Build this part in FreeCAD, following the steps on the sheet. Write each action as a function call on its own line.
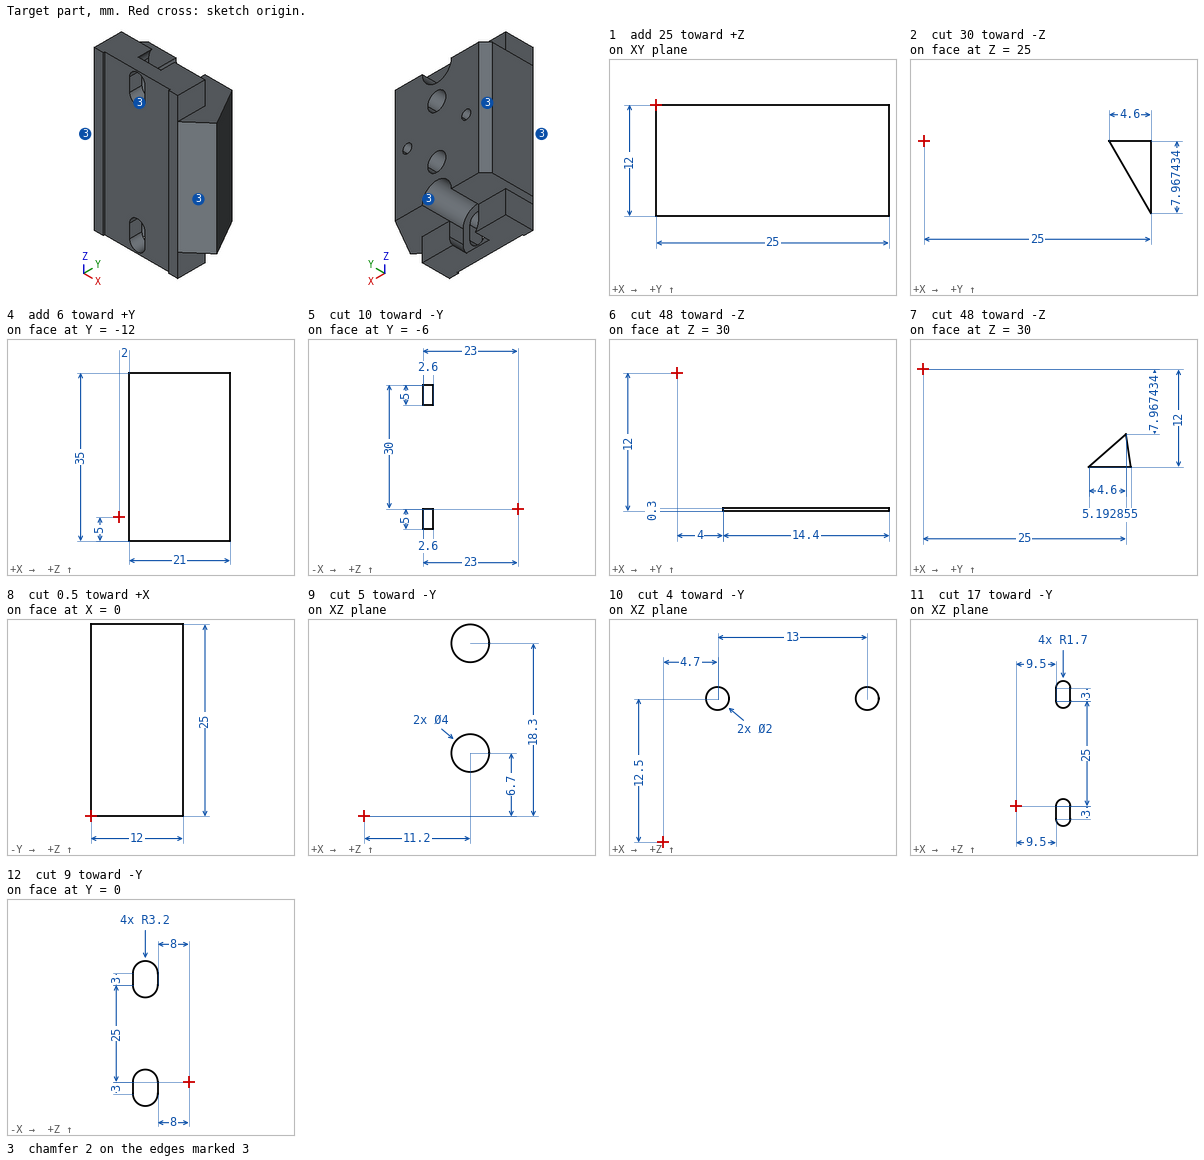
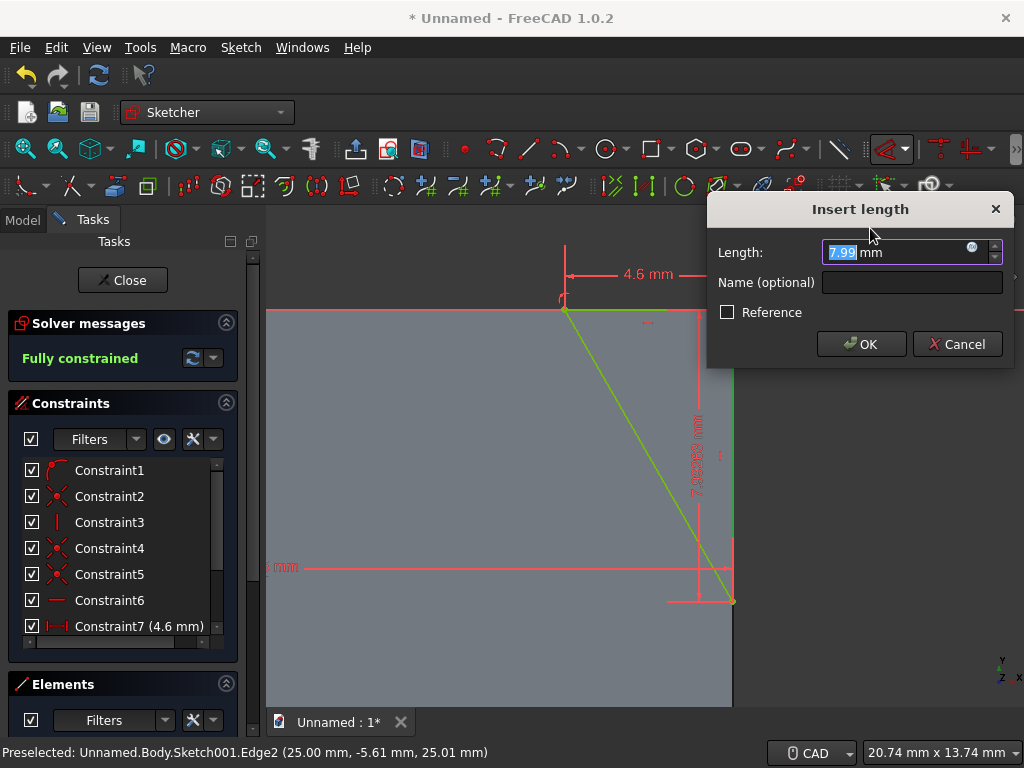
text(7.967434)
key(Return)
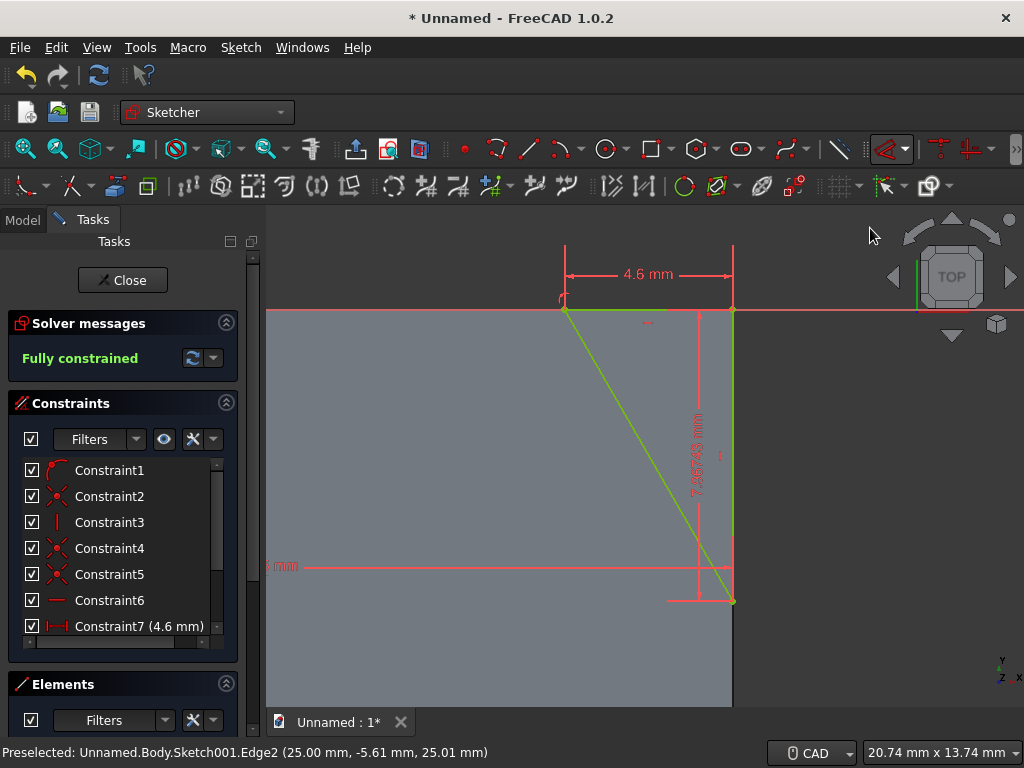
click(123, 280)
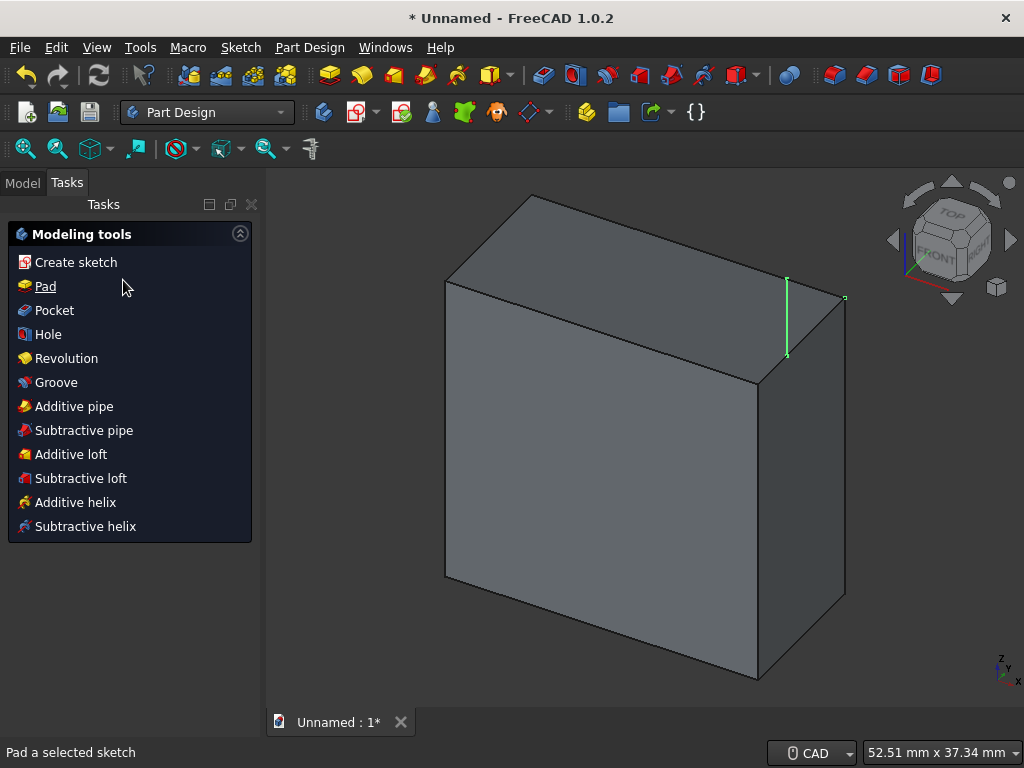
click(544, 76)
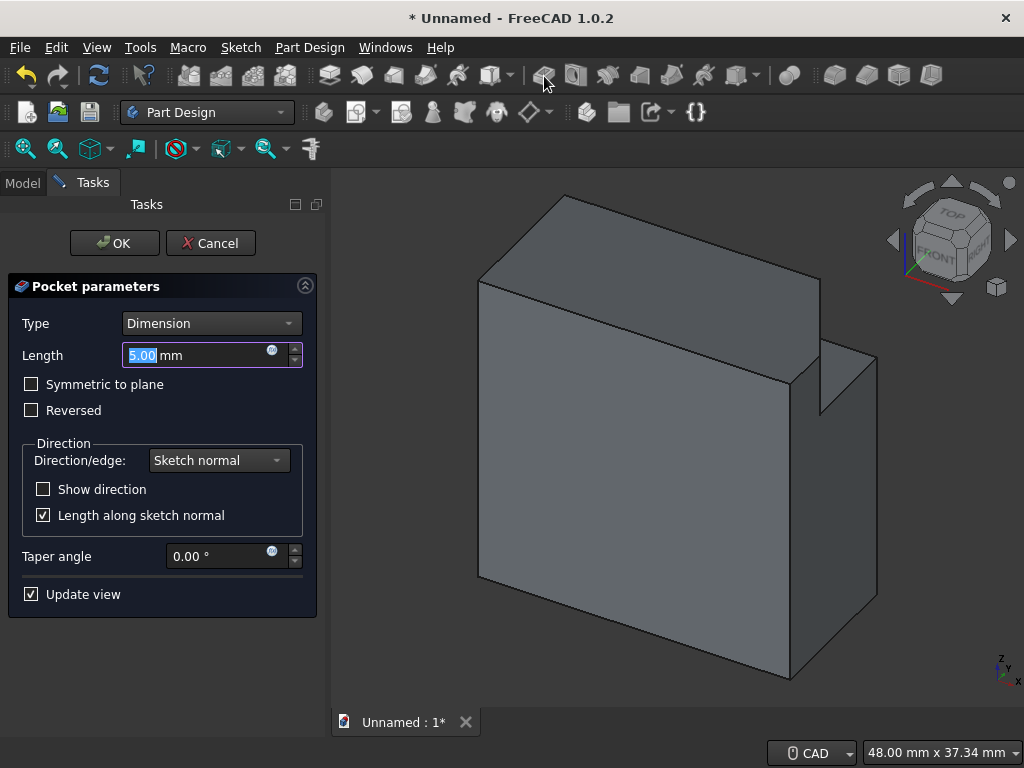
text(30)
key(Tab)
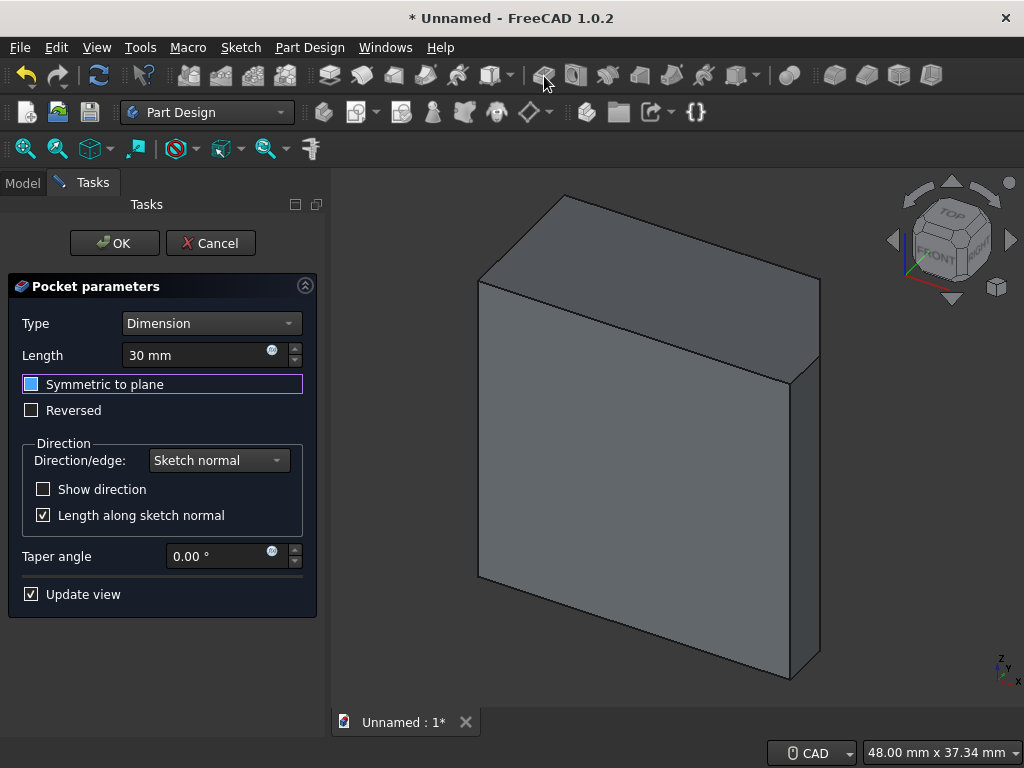
click(115, 243)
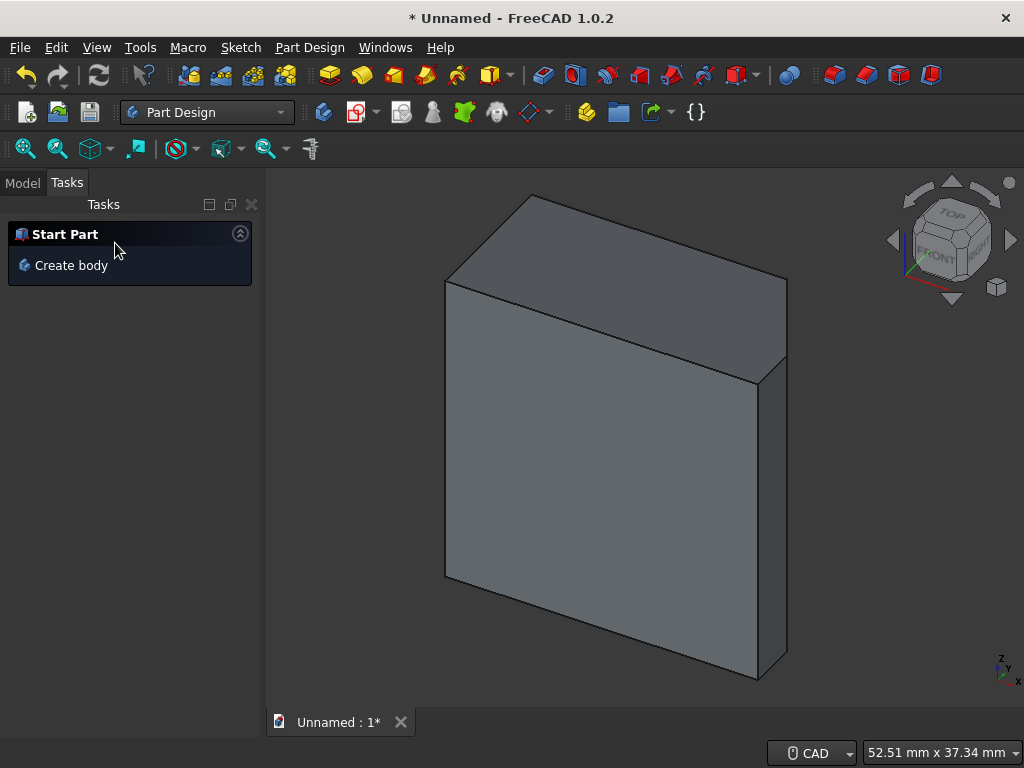
click(758, 531)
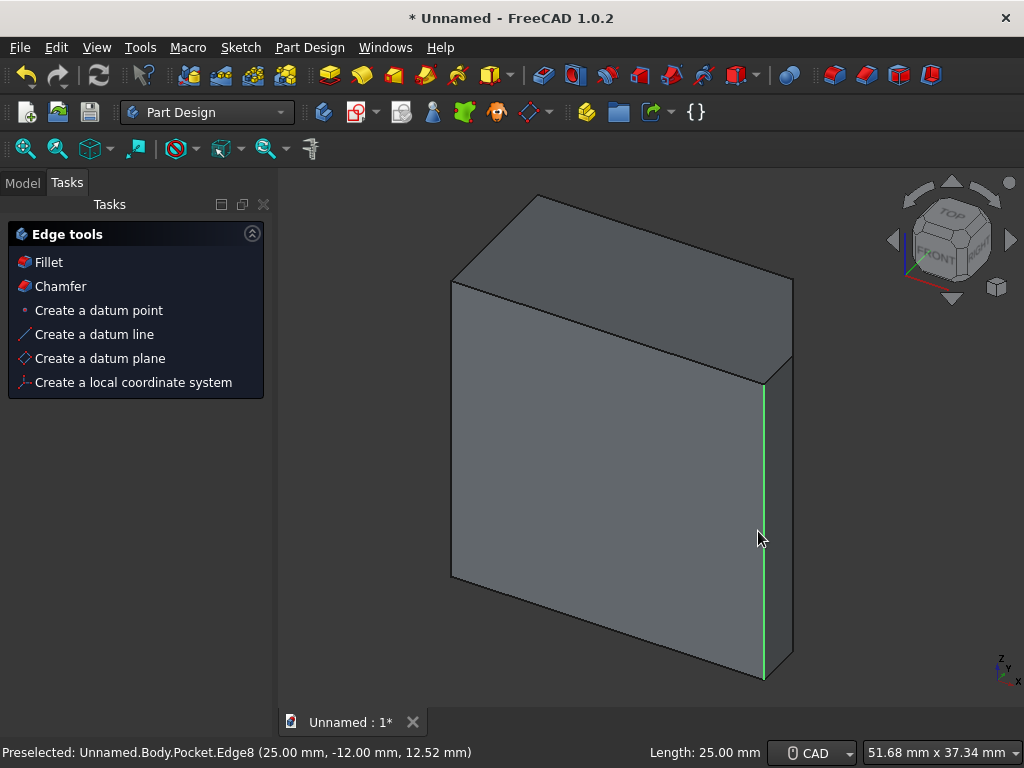
key(0)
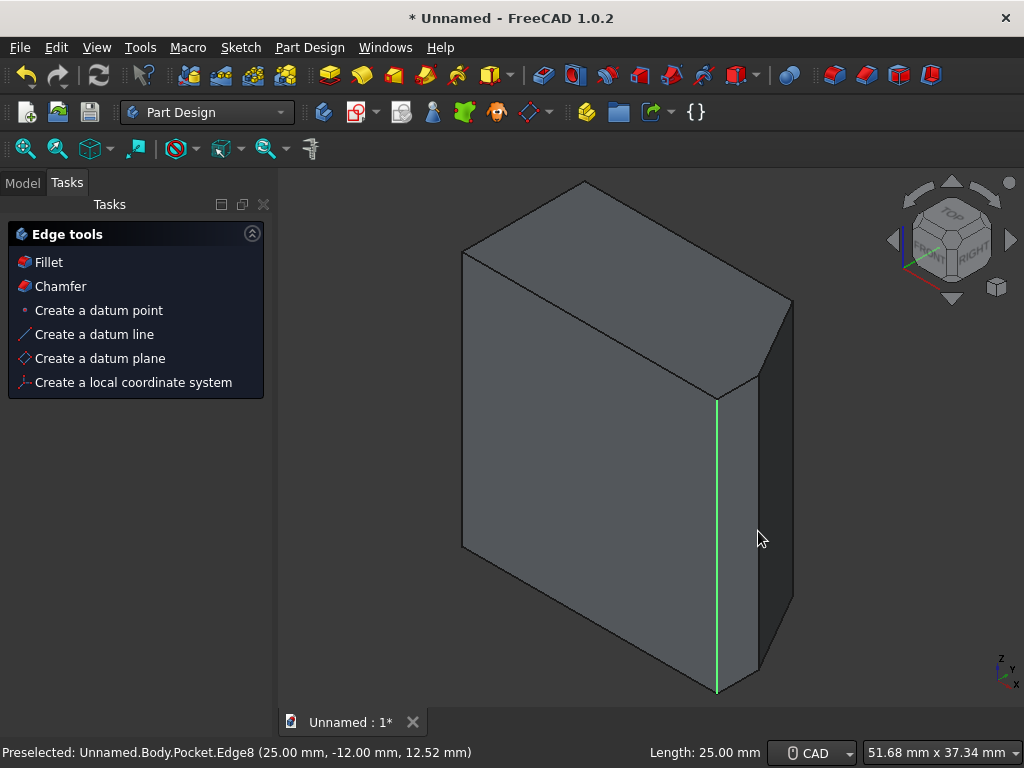
key(2)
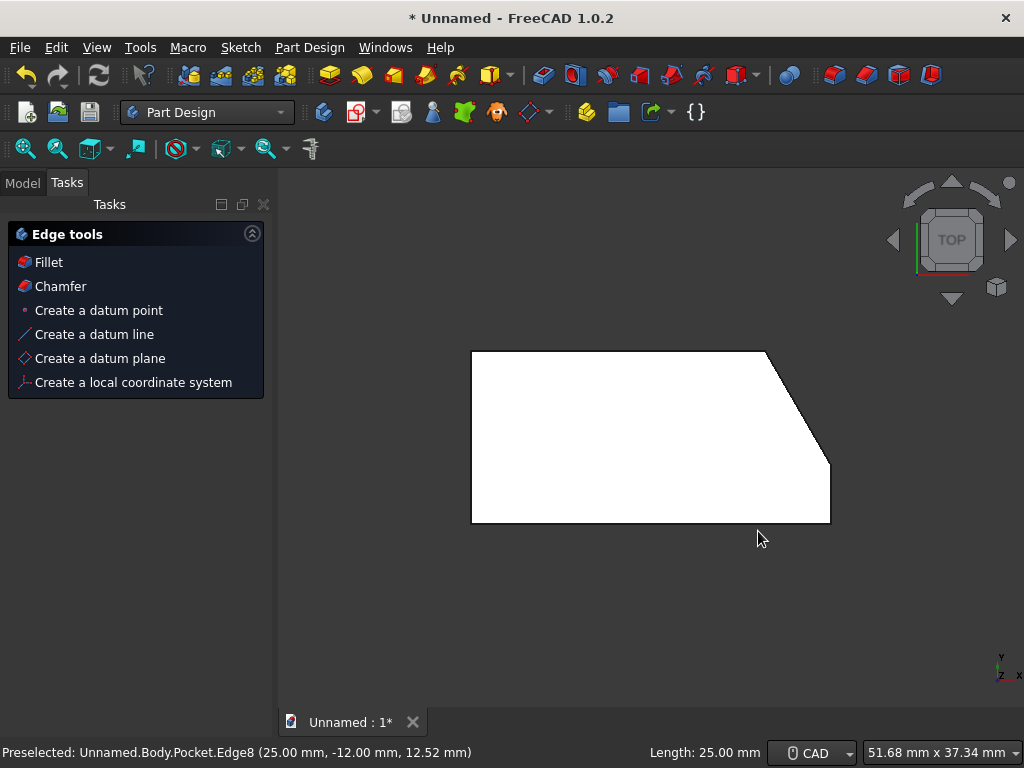
key(1)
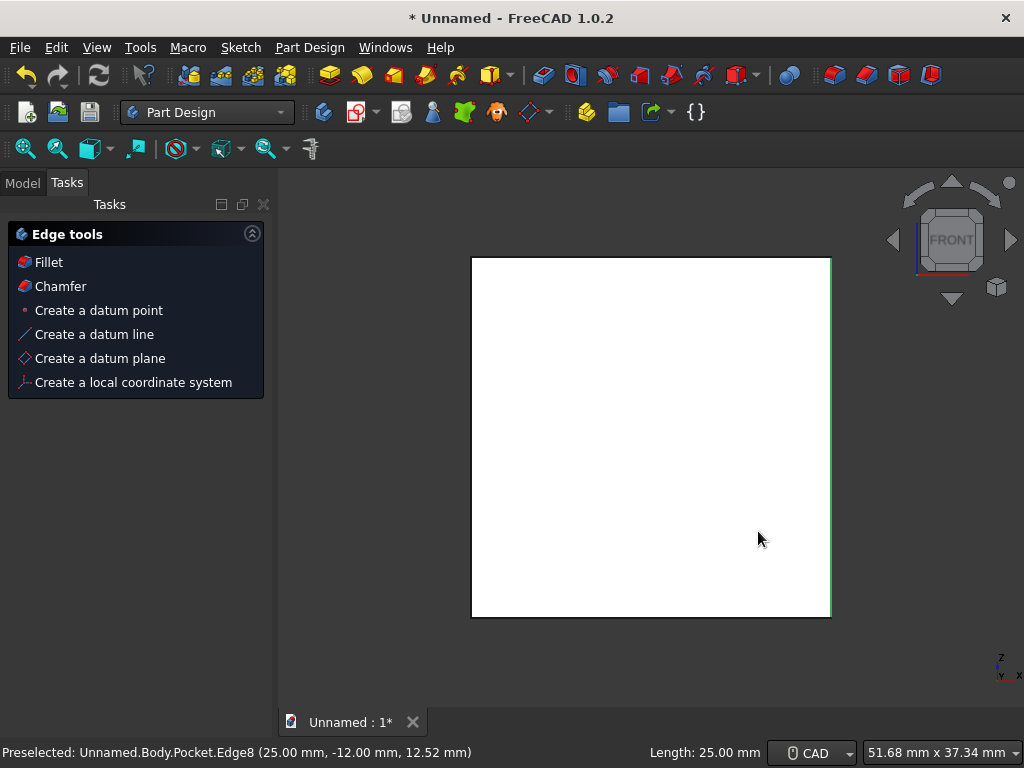
click(471, 437, ctrl)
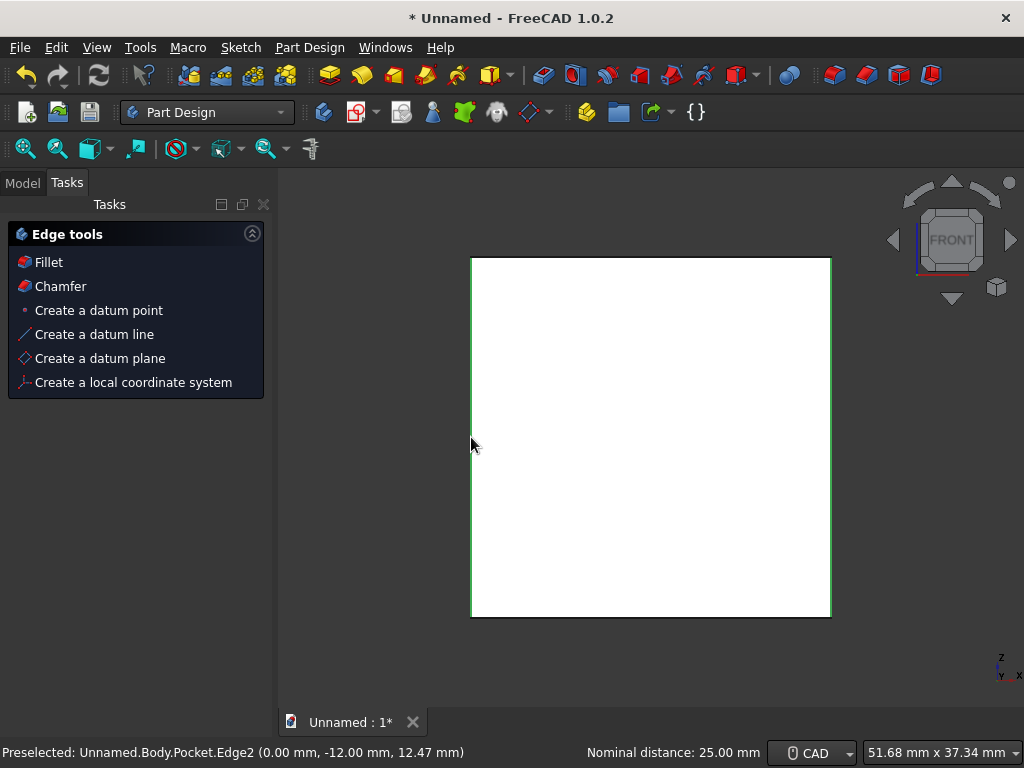
key(3)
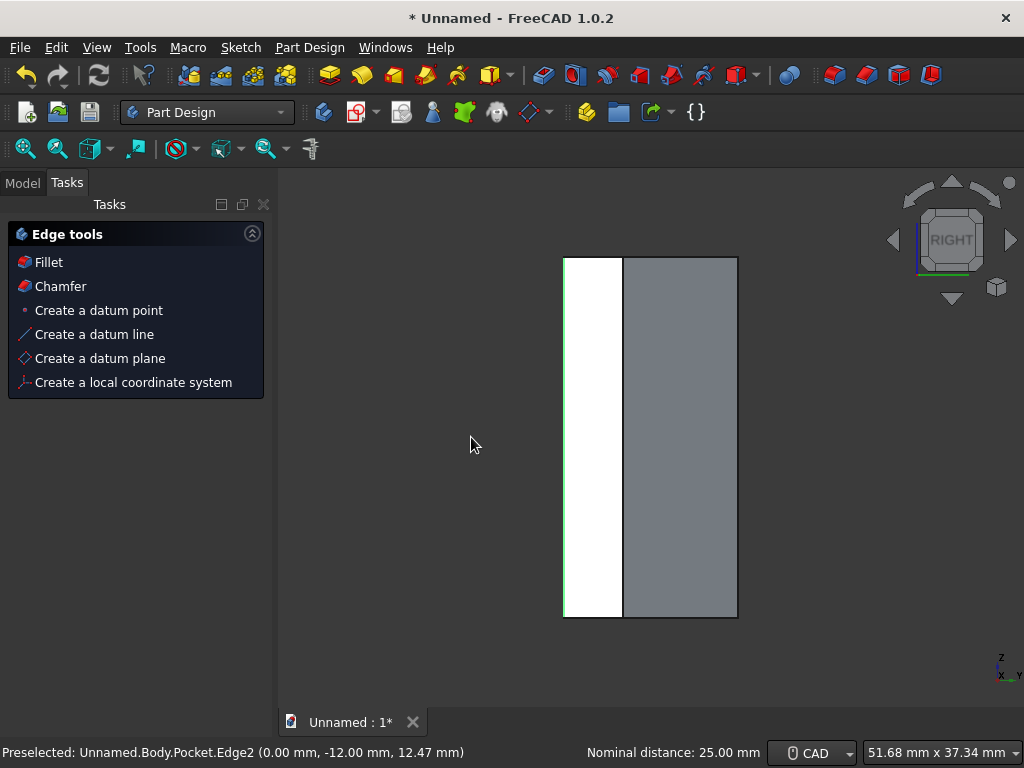
key(5)